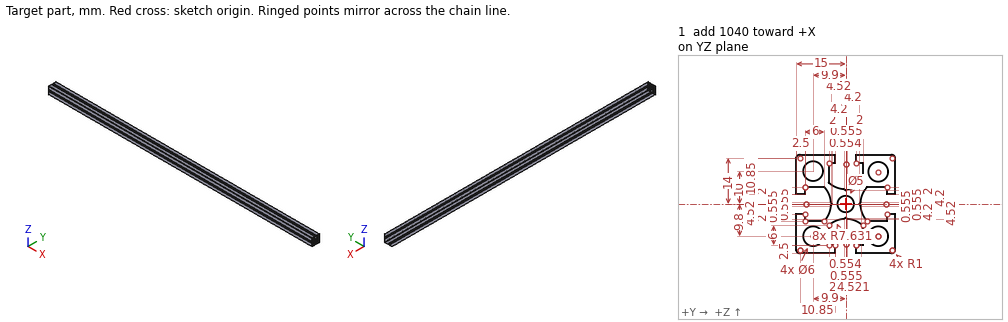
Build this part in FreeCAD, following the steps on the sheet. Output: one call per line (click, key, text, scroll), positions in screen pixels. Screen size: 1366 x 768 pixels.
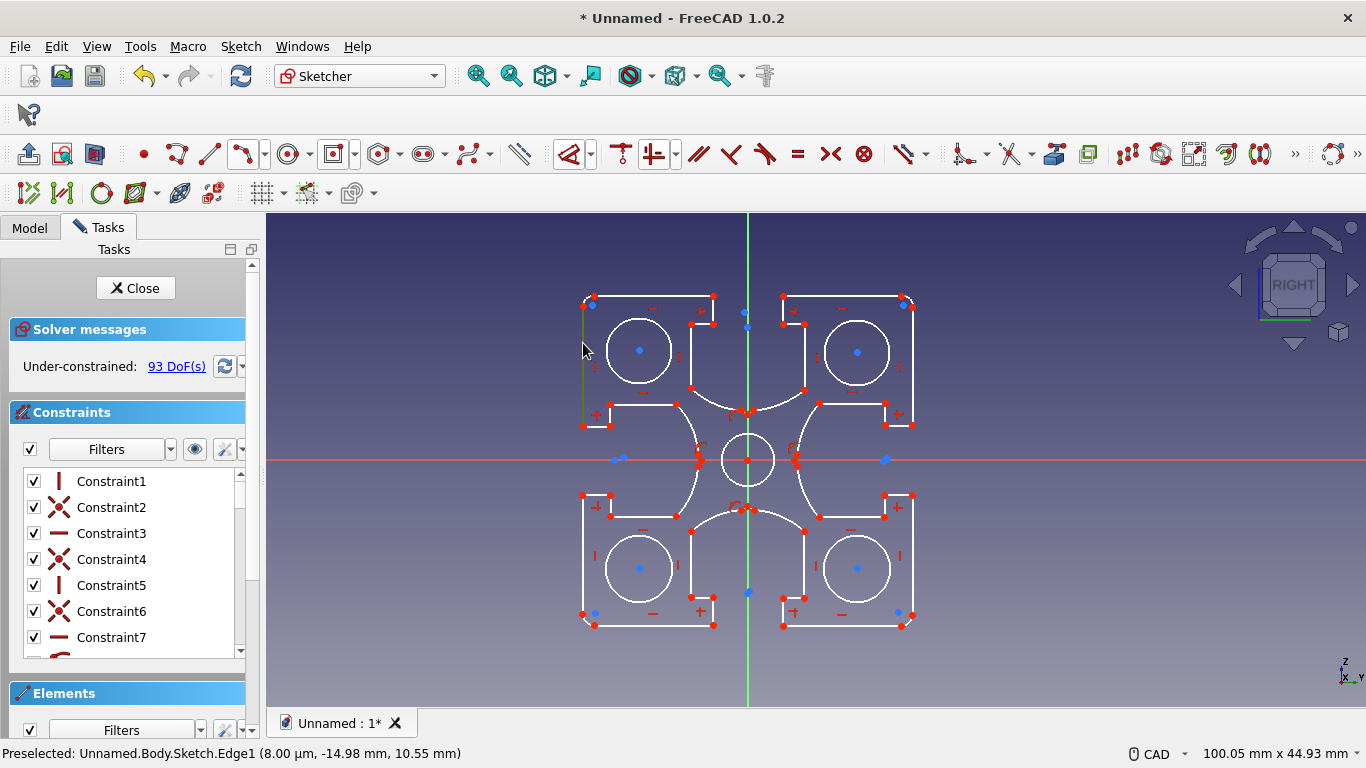
scroll(586, 299, up, 3)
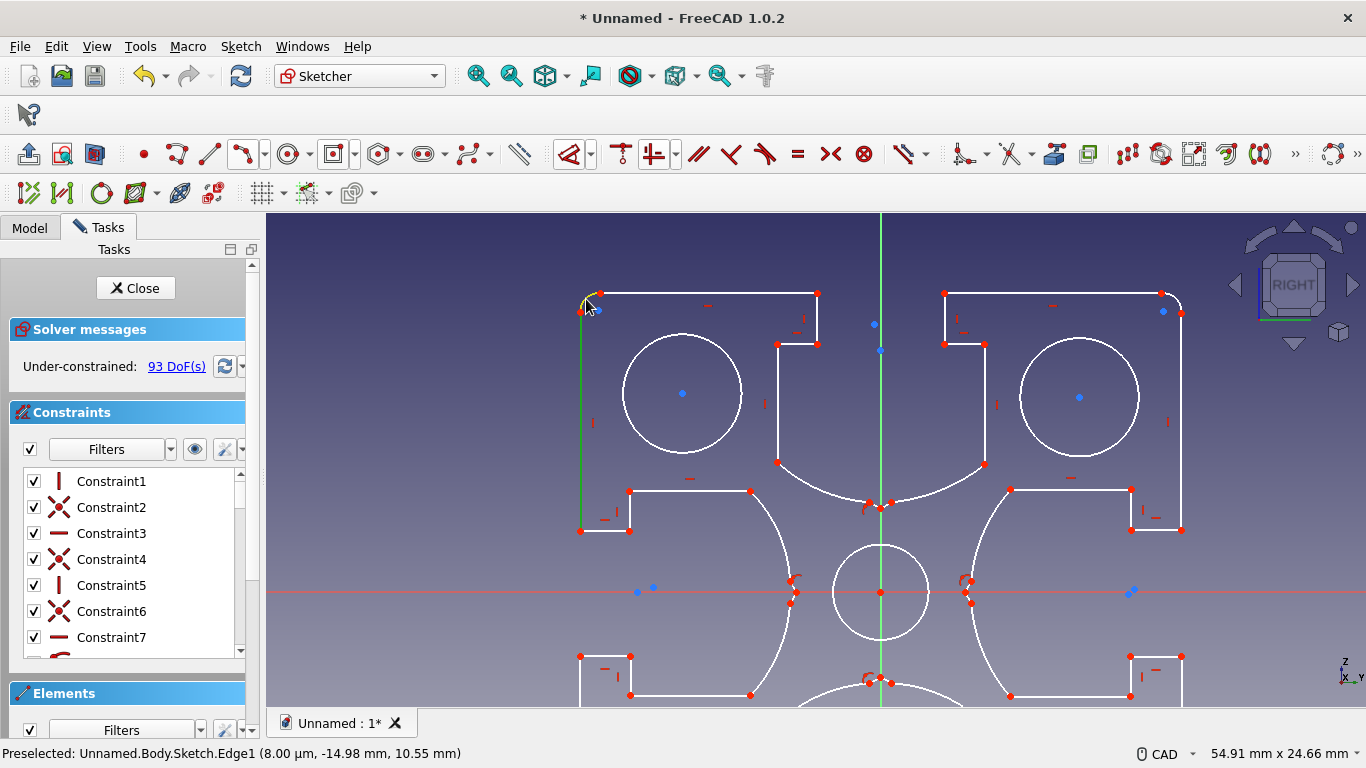
click(586, 298)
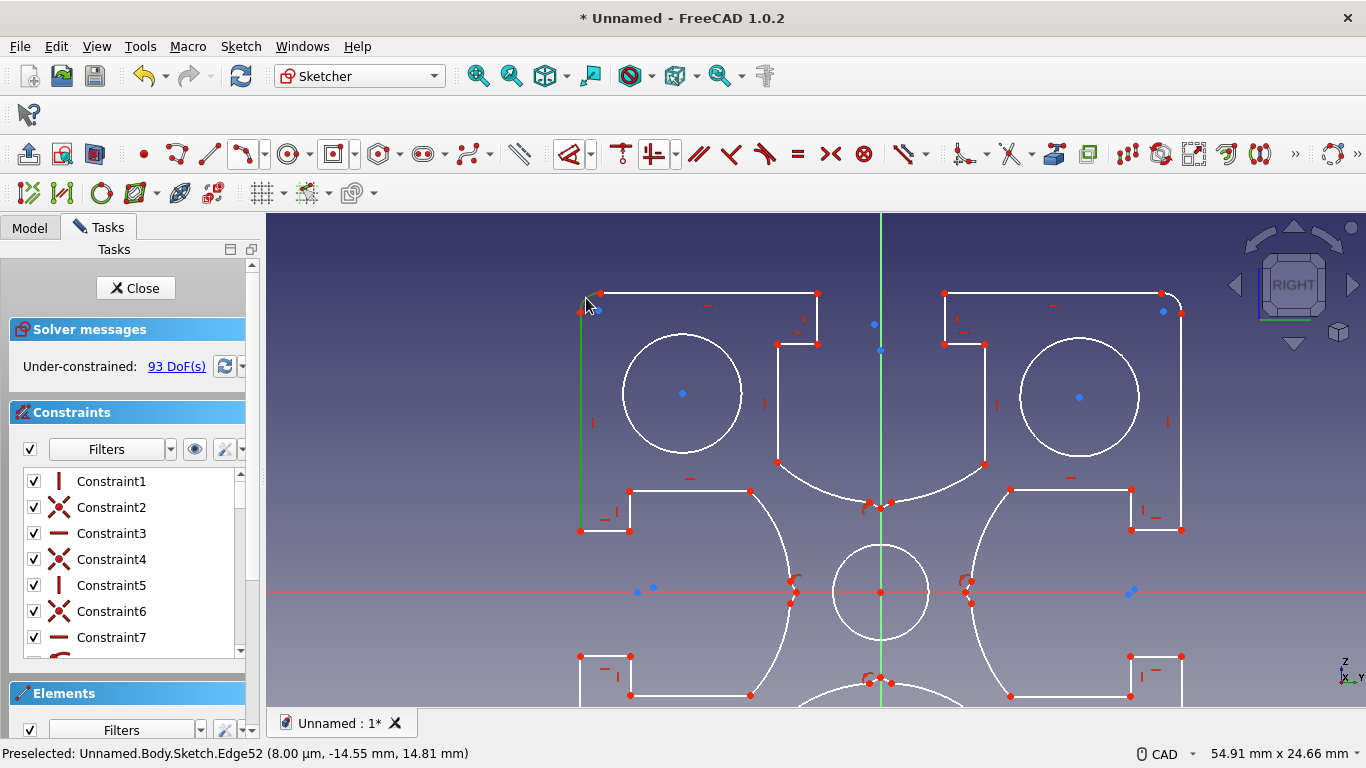
key(t)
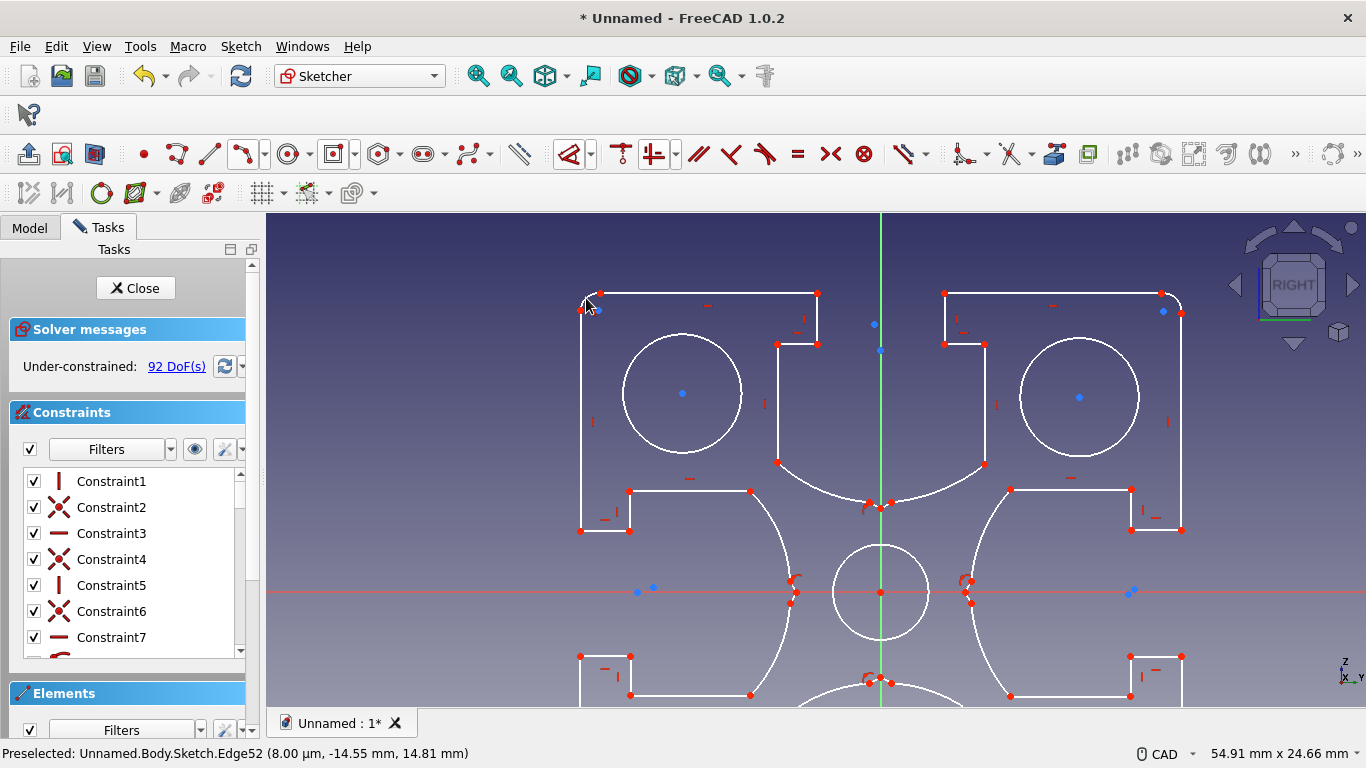
scroll(585, 299, down, 3)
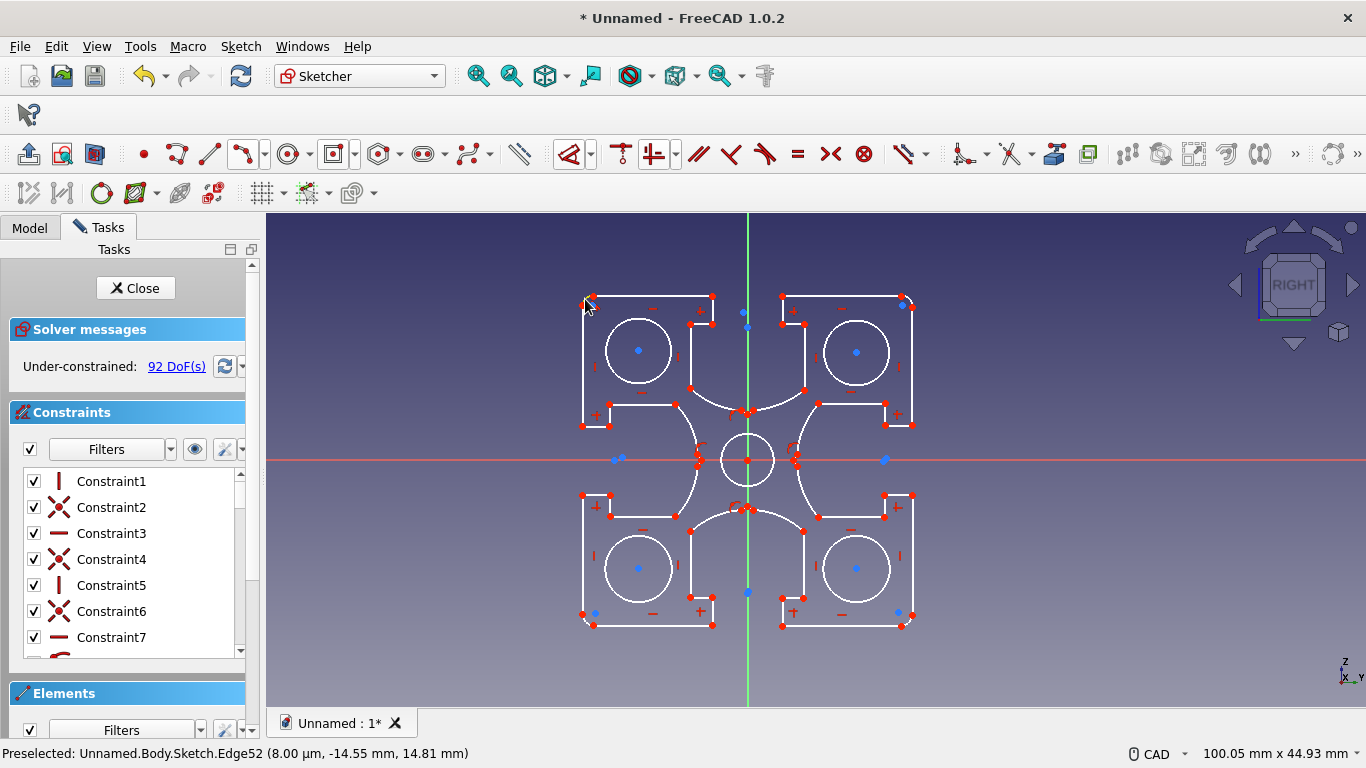
click(583, 531)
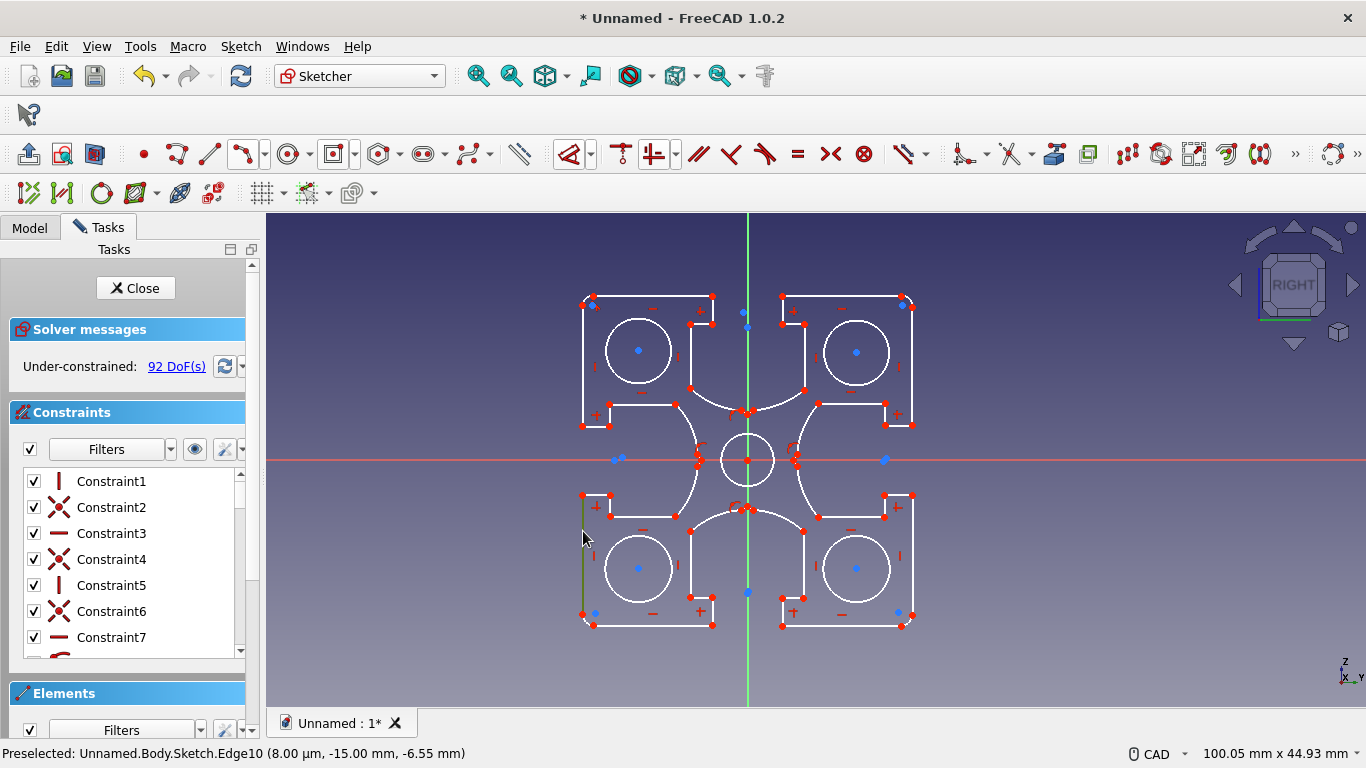
scroll(586, 622, up, 3)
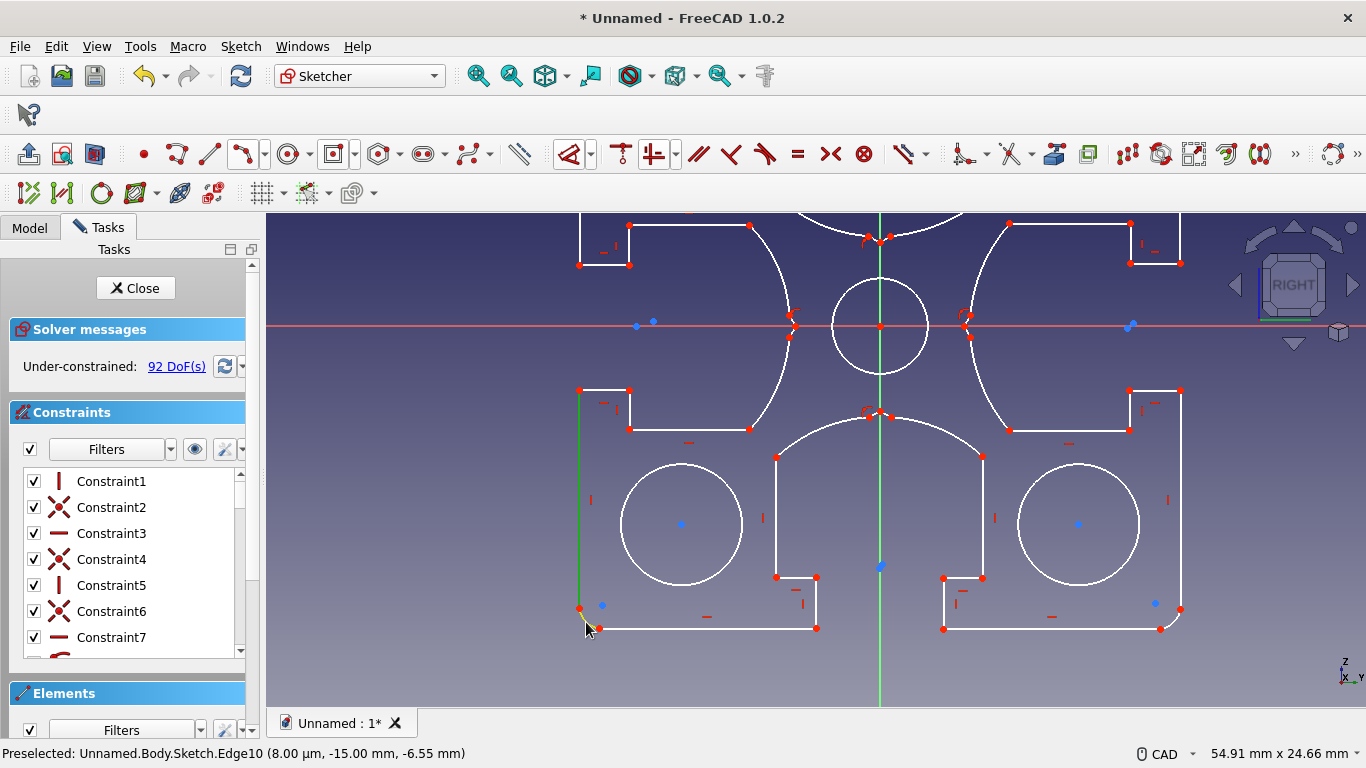
click(586, 622)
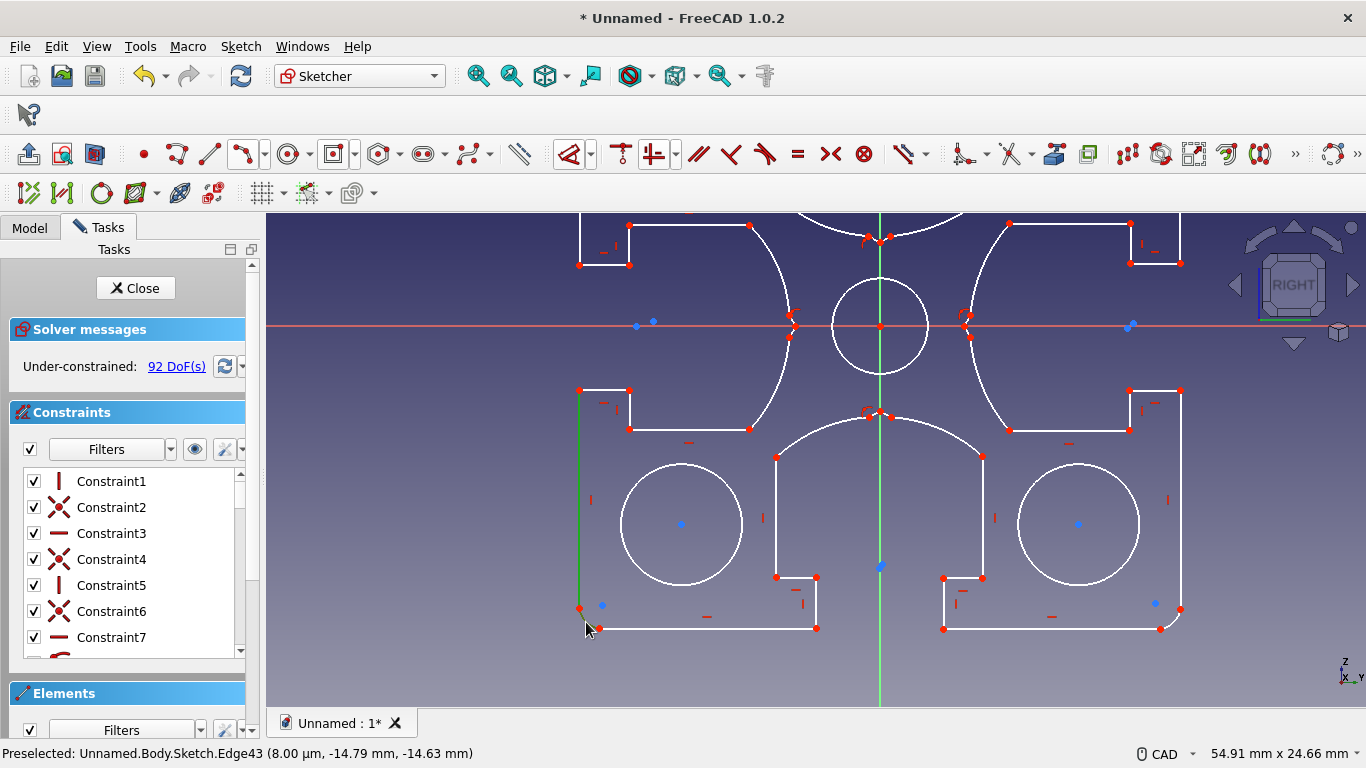
click(765, 154)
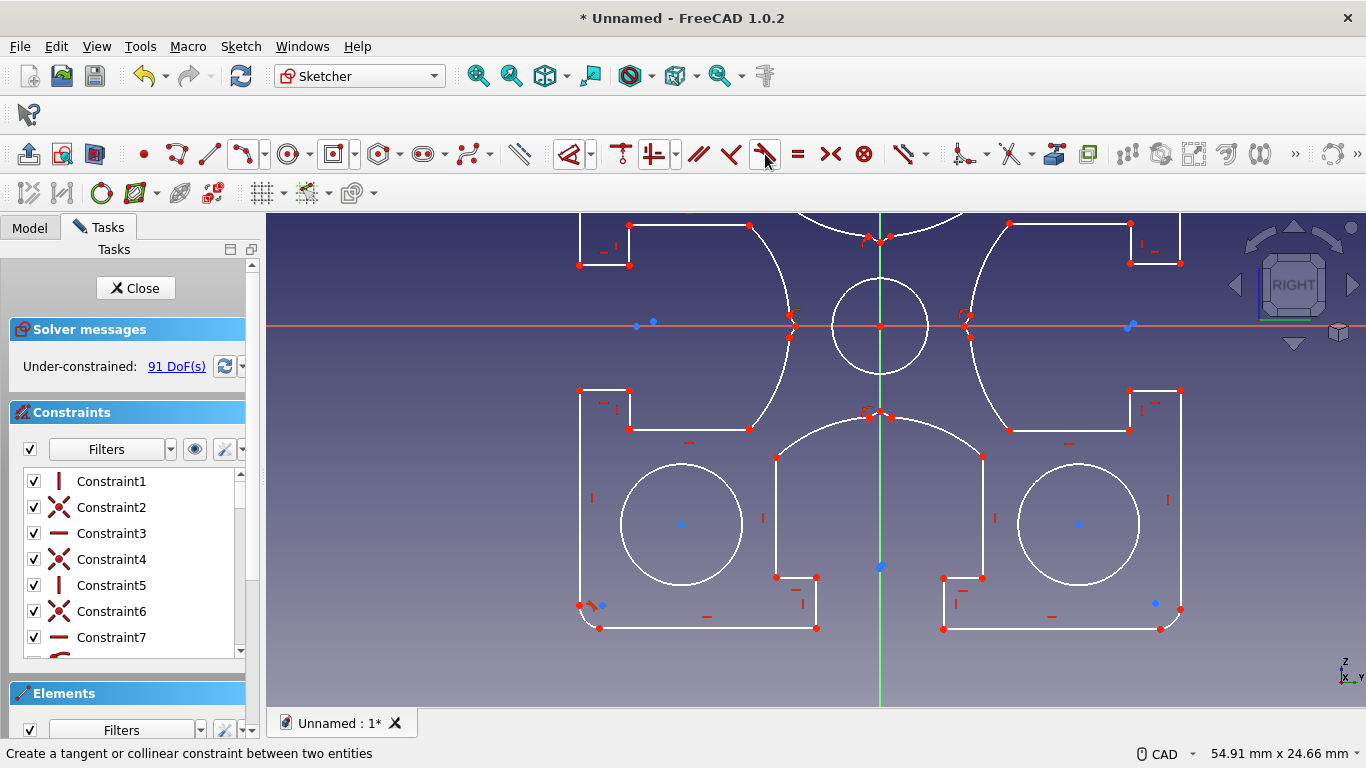
click(665, 628)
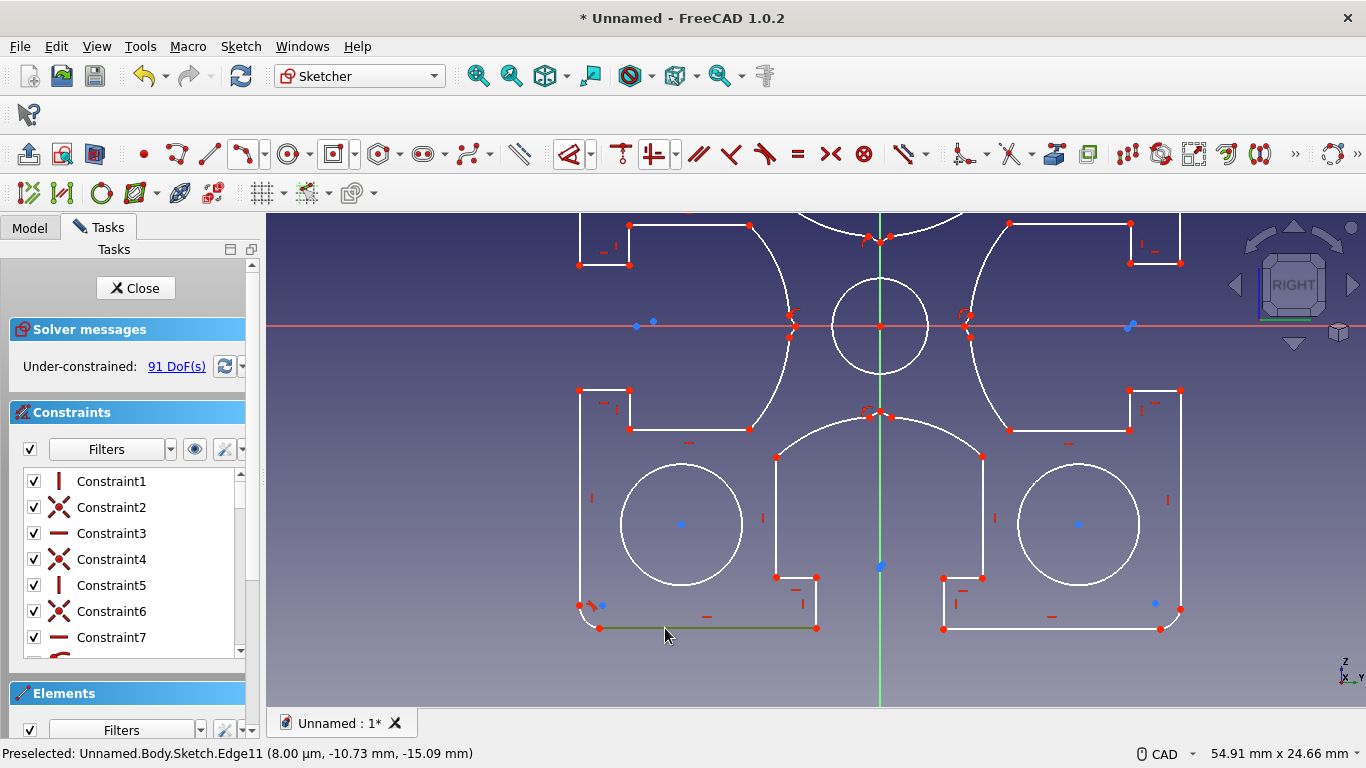
scroll(582, 615, up, 2)